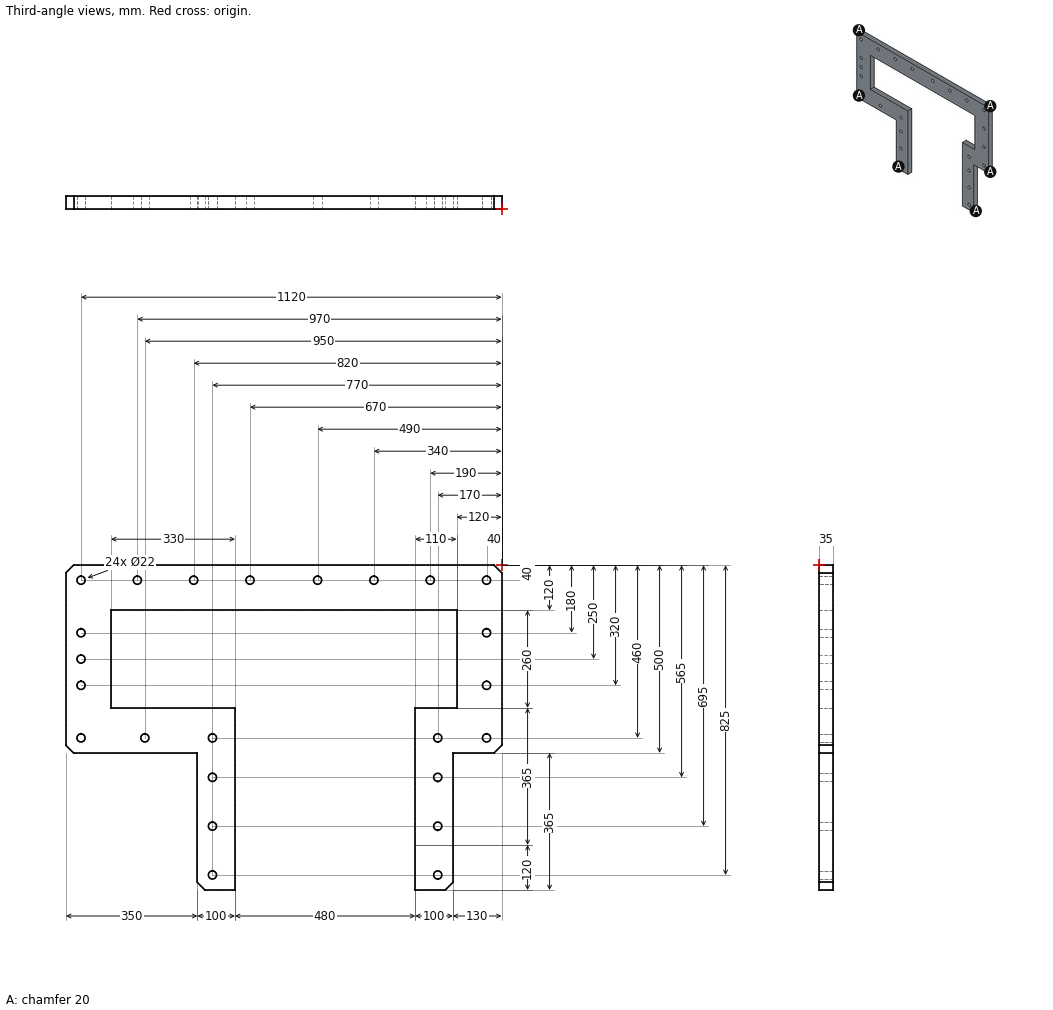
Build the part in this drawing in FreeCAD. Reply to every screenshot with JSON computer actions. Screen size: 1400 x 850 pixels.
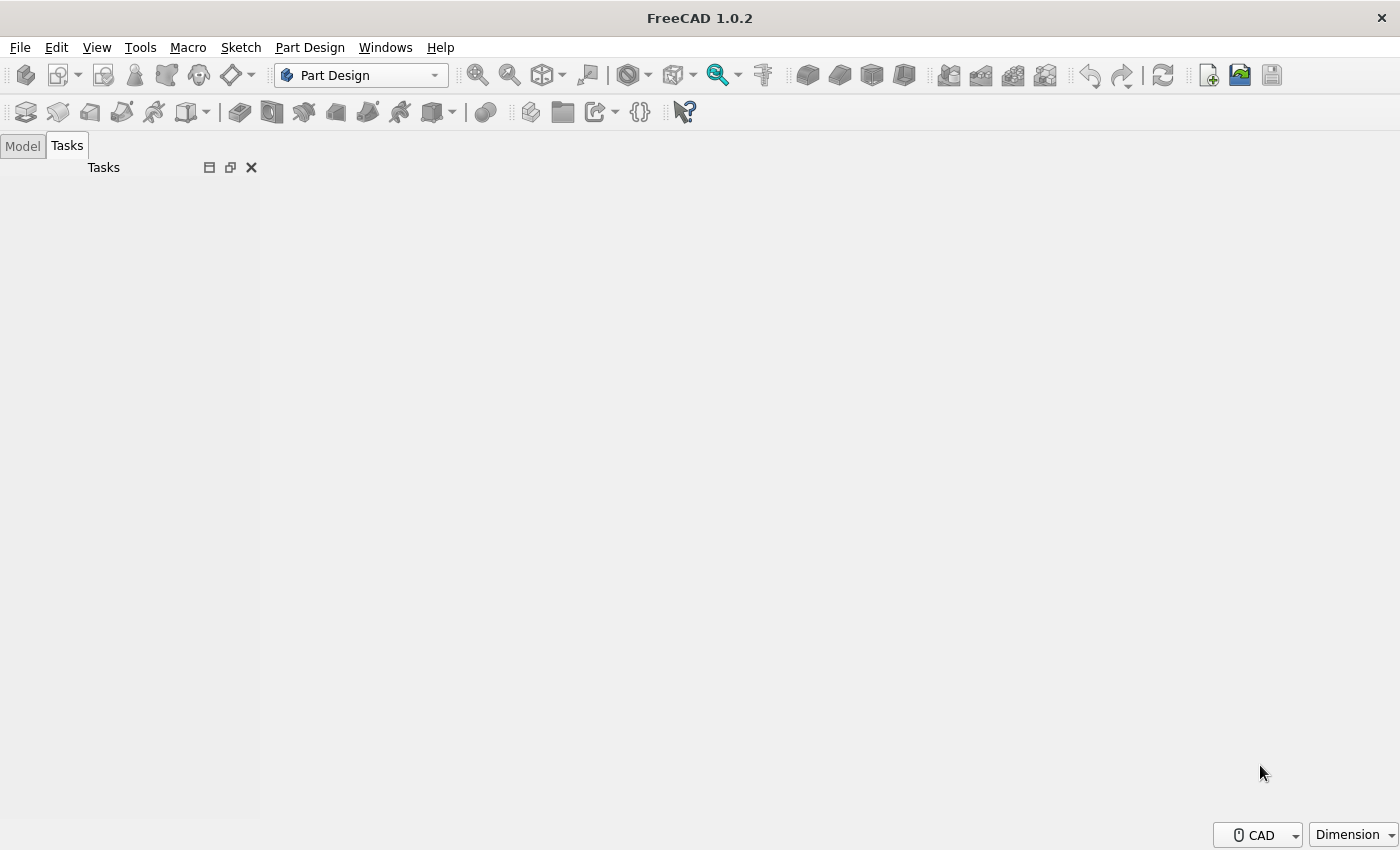
{"action": "key", "text": "ctrl+n"}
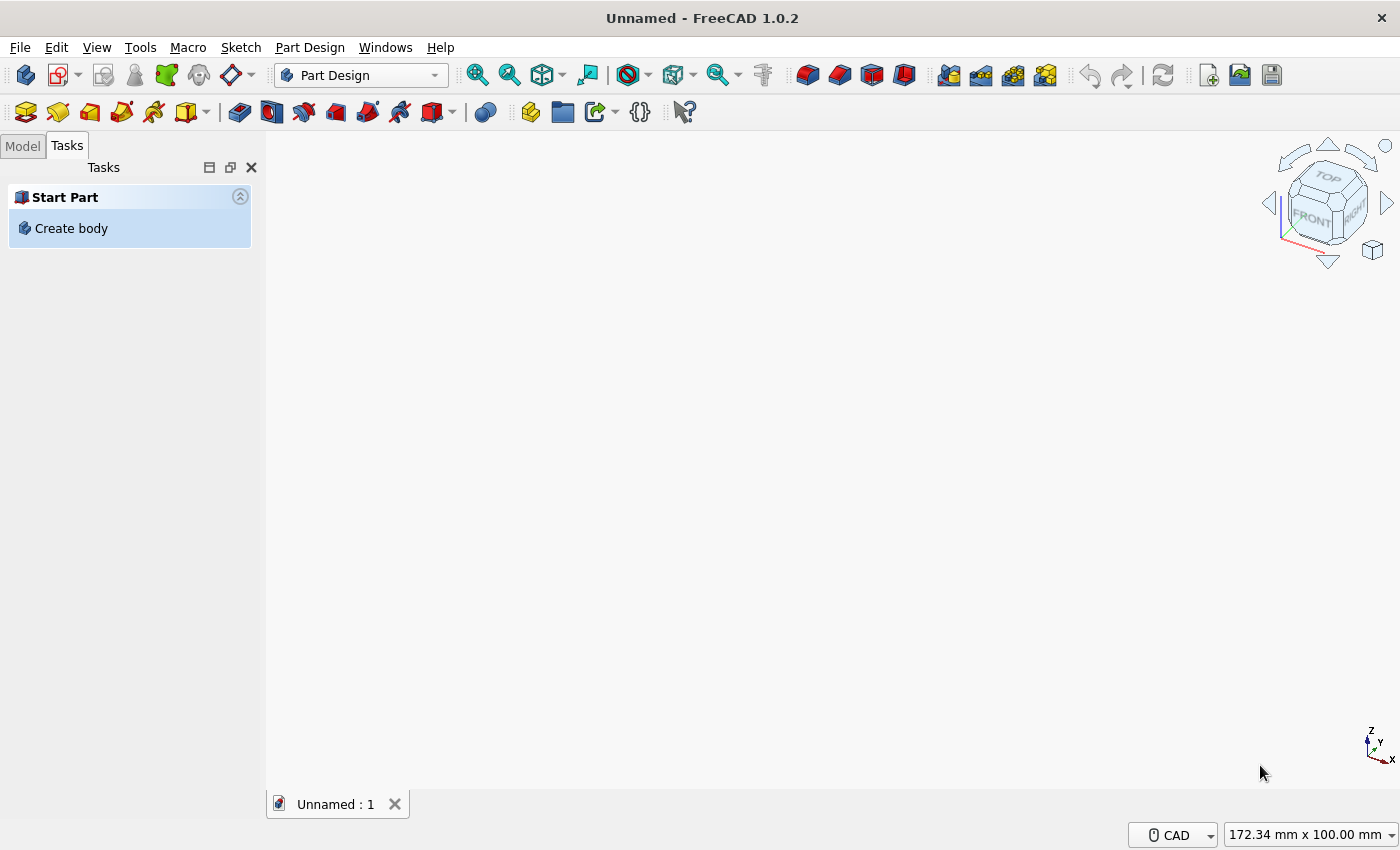
{"action": "left_click", "coordinate": [58, 76]}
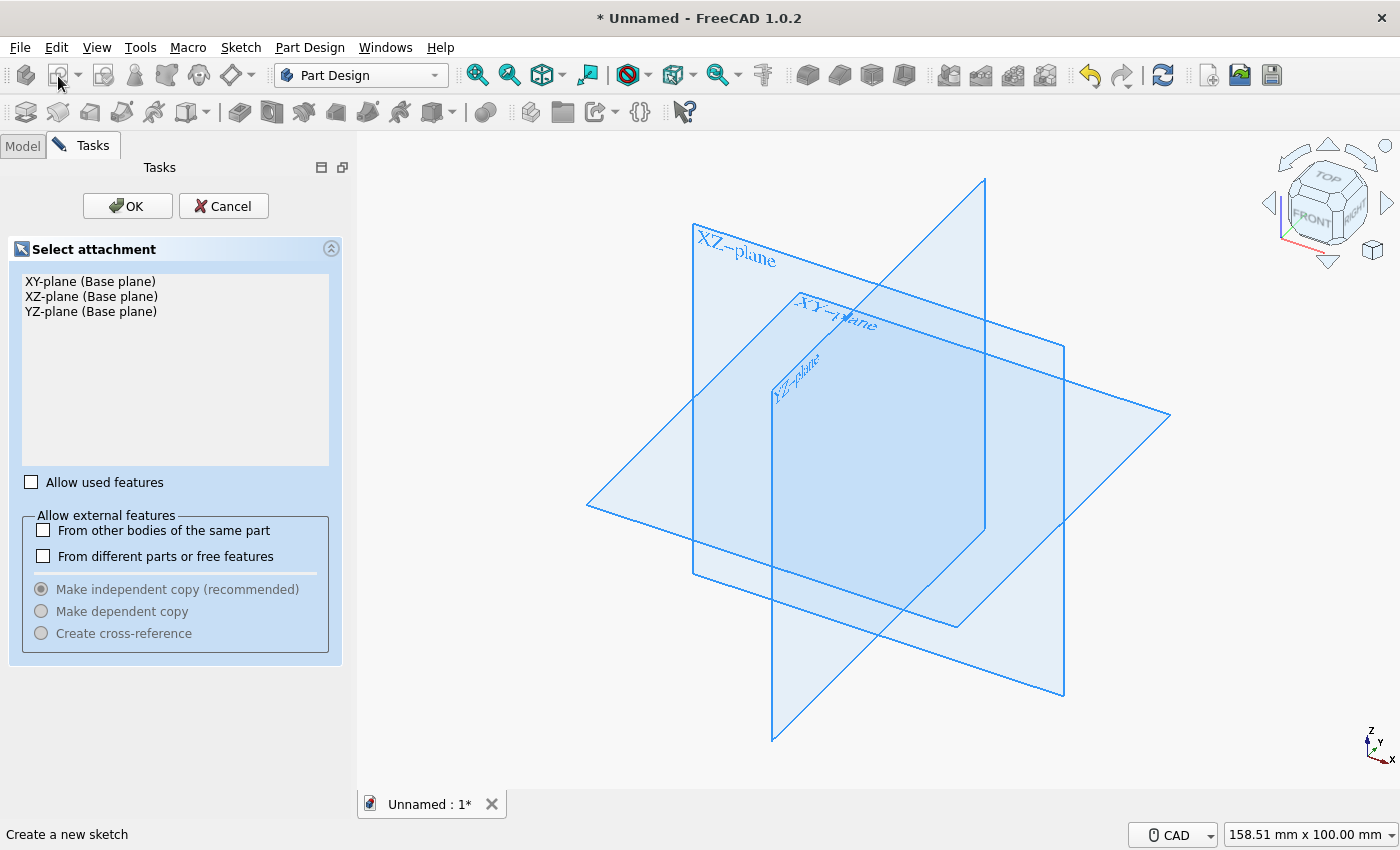
{"action": "left_click", "coordinate": [82, 296]}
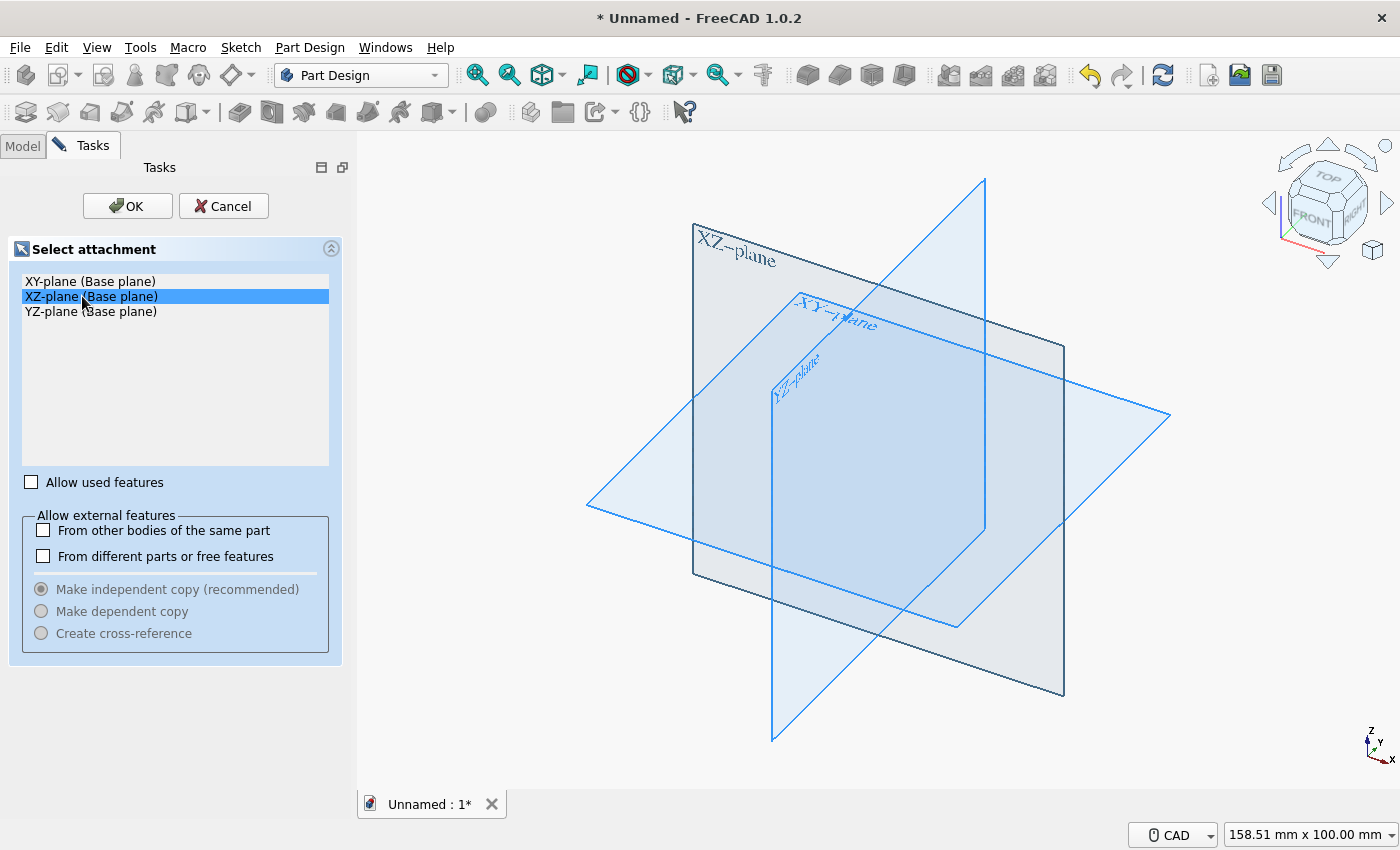
{"action": "left_click", "coordinate": [128, 206]}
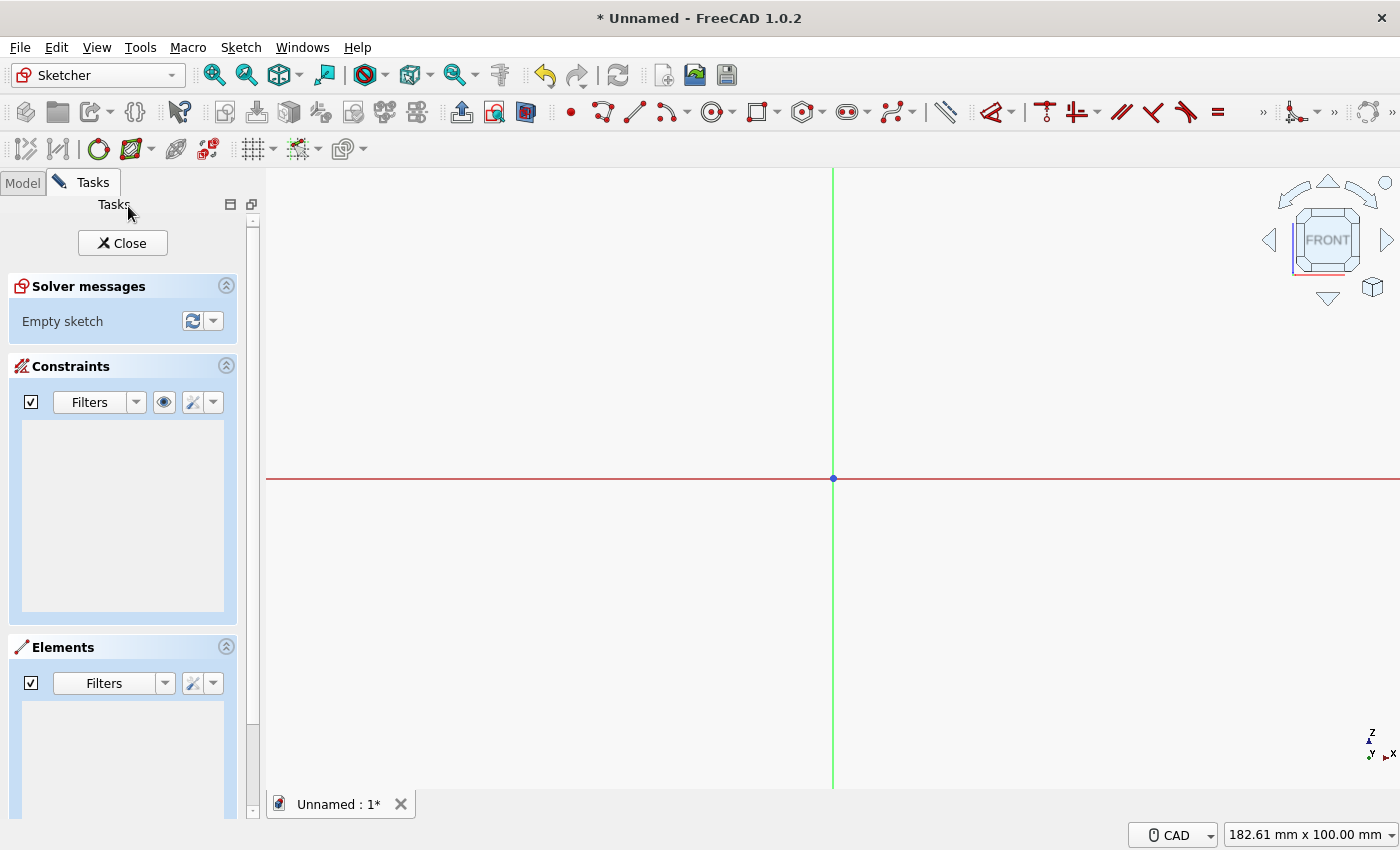
{"action": "scroll", "coordinate": [1048, 263], "scroll_direction": "down", "scroll_amount": 13}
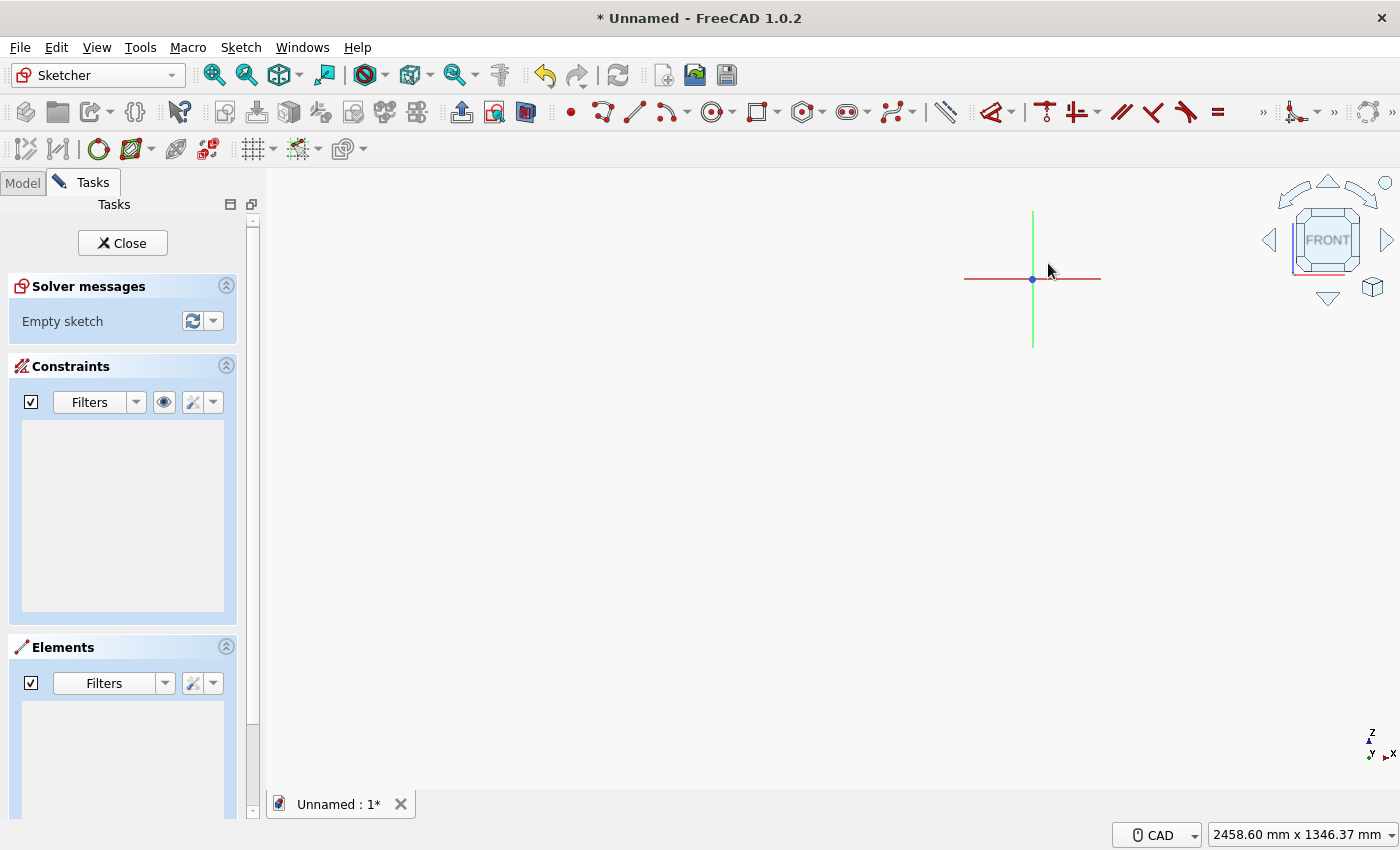
{"action": "left_click", "coordinate": [604, 112]}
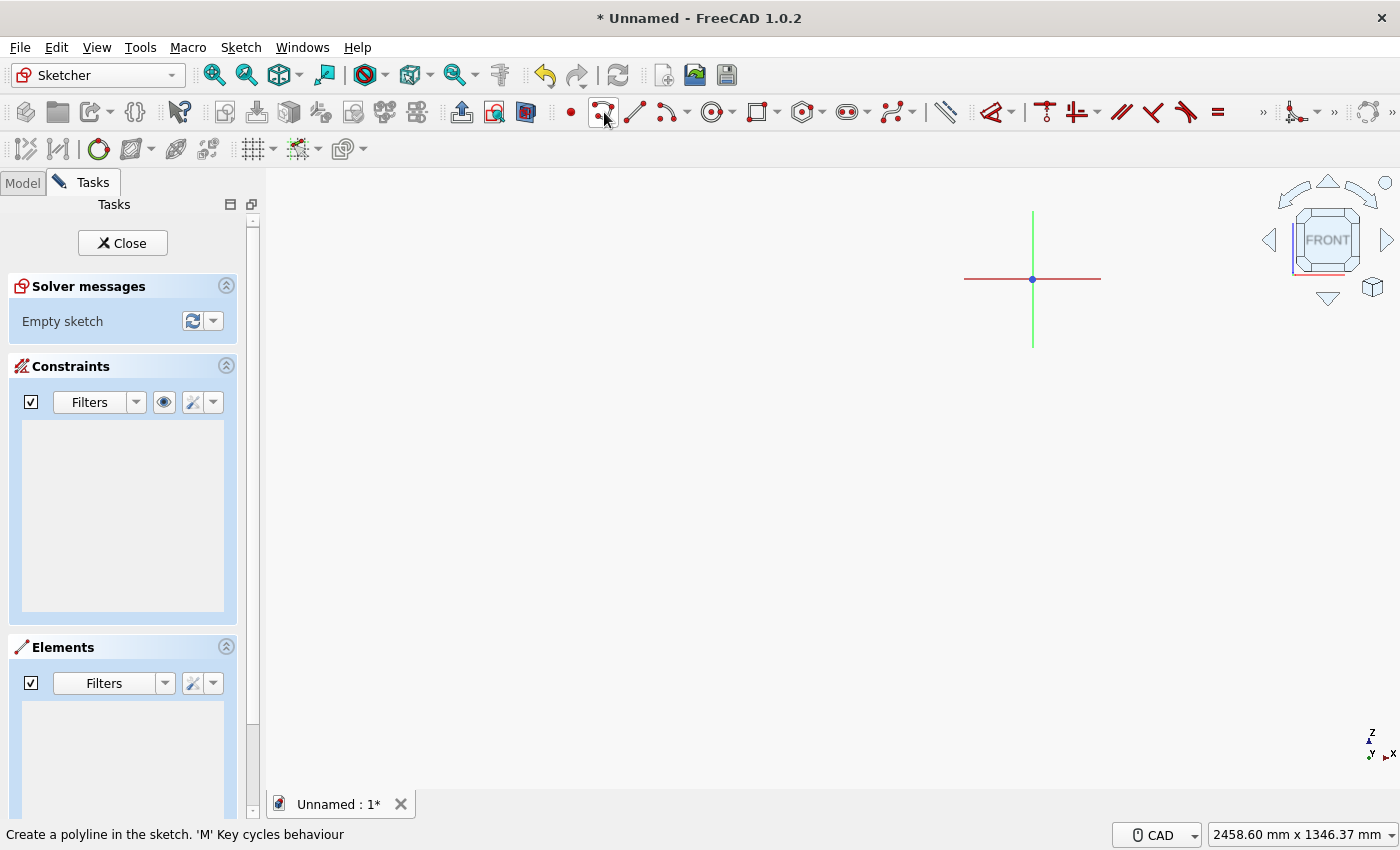
{"action": "left_click", "coordinate": [1033, 279]}
{"action": "left_click", "coordinate": [1024, 510]}
{"action": "left_click", "coordinate": [973, 510]}
{"action": "left_click", "coordinate": [973, 678]}
{"action": "left_click", "coordinate": [927, 678]}
{"action": "left_click", "coordinate": [927, 623]}
{"action": "left_click", "coordinate": [705, 623]}
{"action": "left_click", "coordinate": [705, 678]}
{"action": "left_click", "coordinate": [659, 678]}
{"action": "left_click", "coordinate": [659, 510]}
{"action": "left_click", "coordinate": [498, 510]}
{"action": "left_click", "coordinate": [498, 288]}
{"action": "left_click", "coordinate": [1033, 279]}
{"action": "key", "text": "Escape"}
{"action": "key", "text": "Escape"}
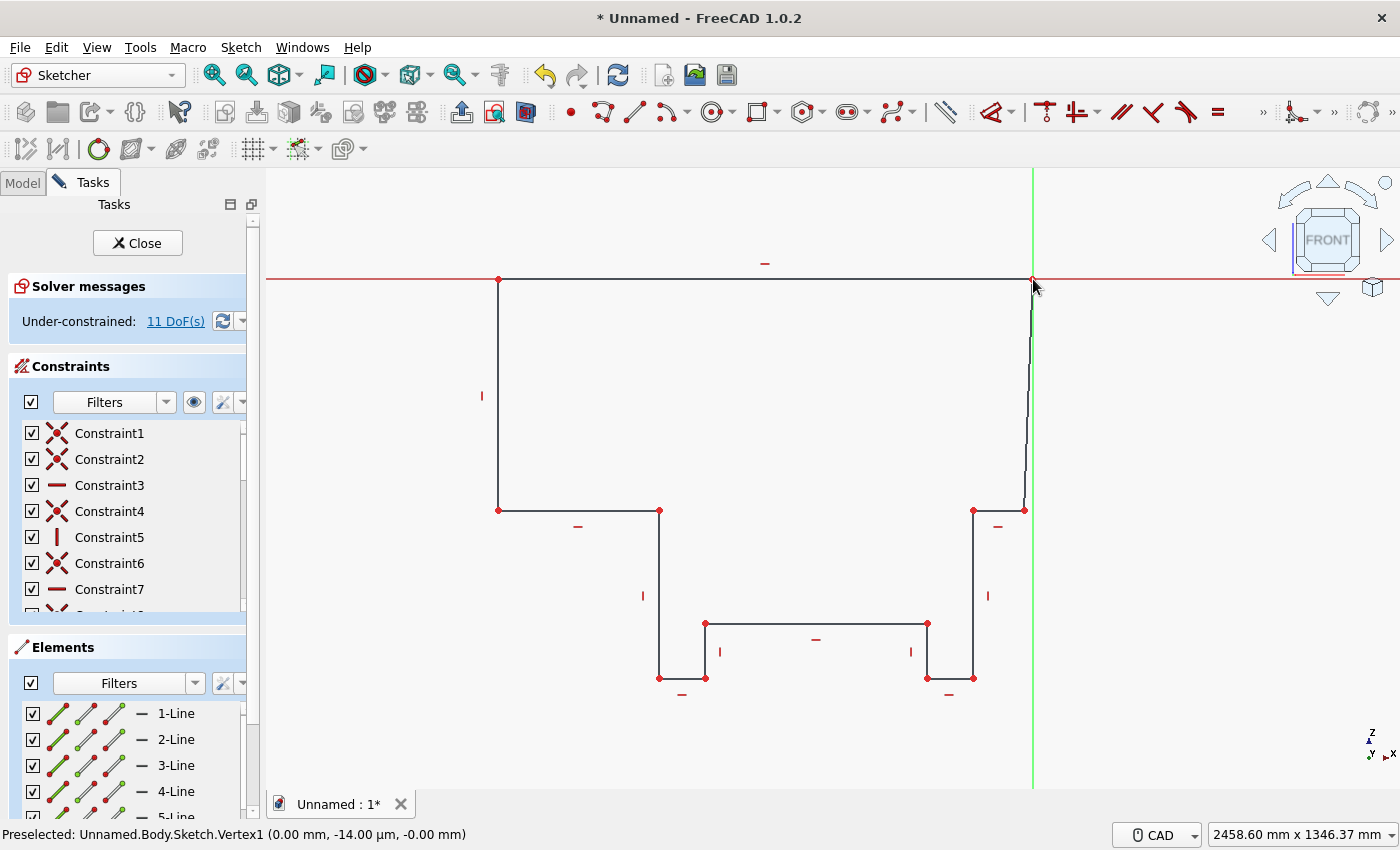
{"action": "left_click", "coordinate": [1030, 349]}